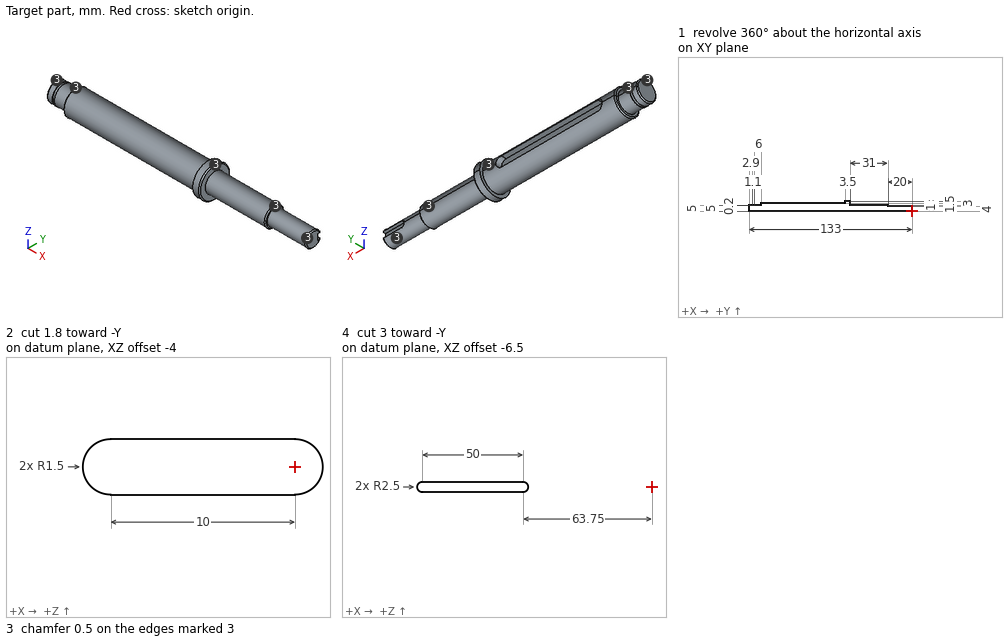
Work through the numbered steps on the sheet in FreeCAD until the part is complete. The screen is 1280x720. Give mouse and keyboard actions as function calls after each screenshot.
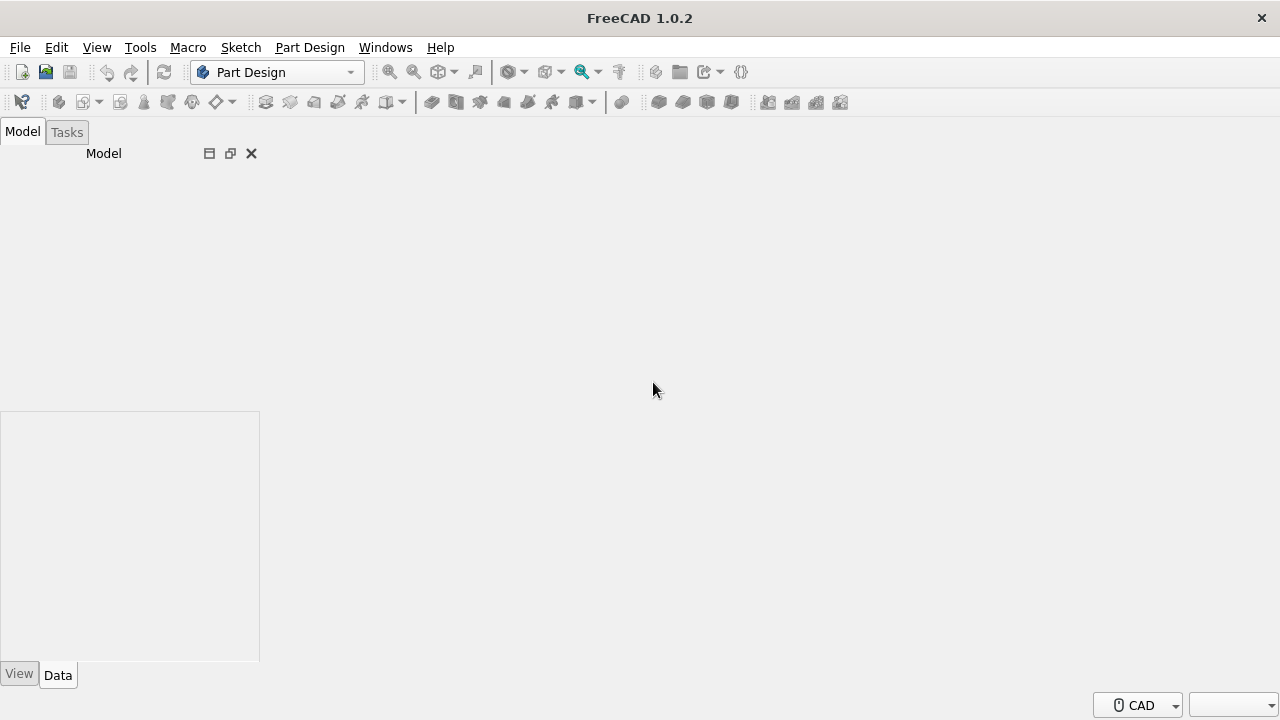
click(22, 72)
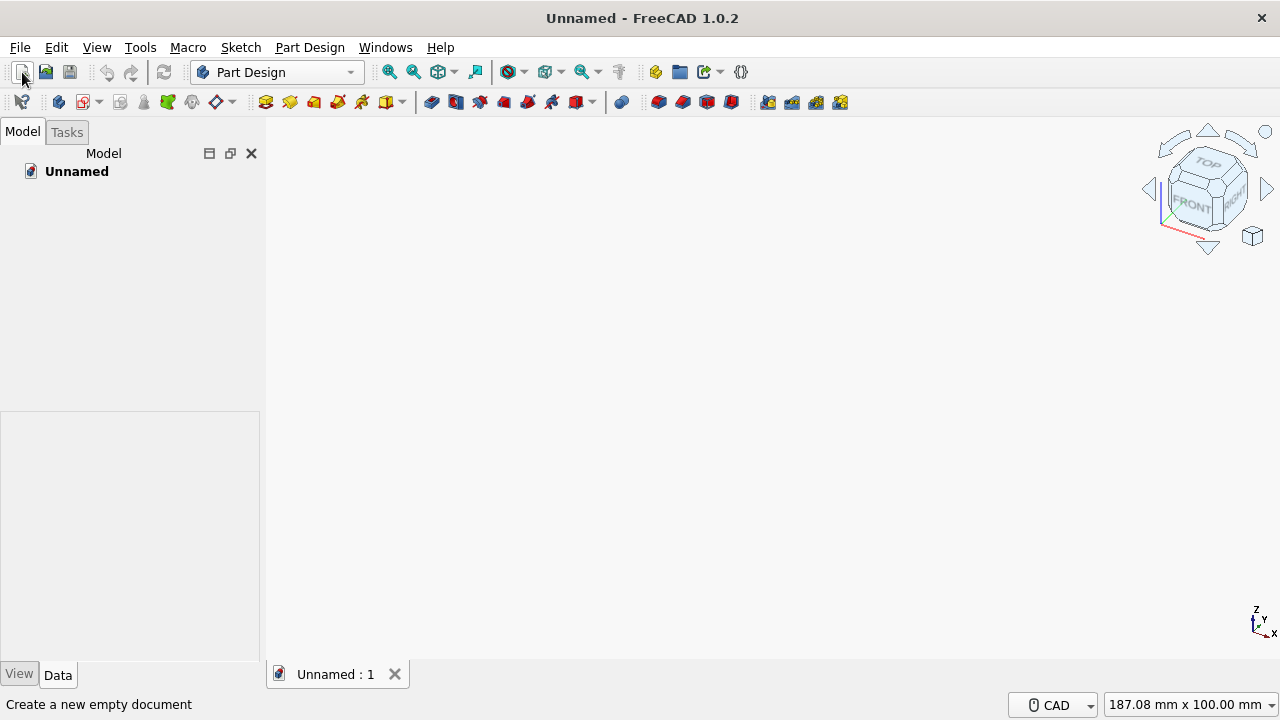
click(84, 102)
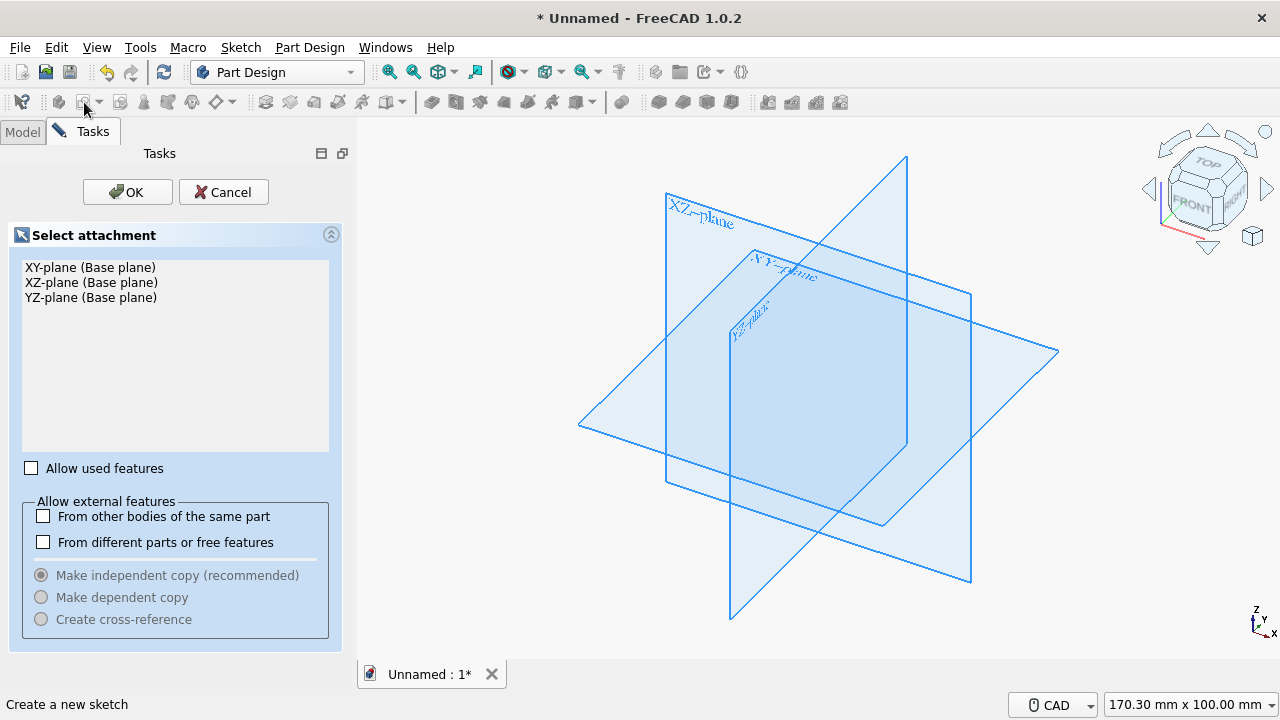
click(82, 268)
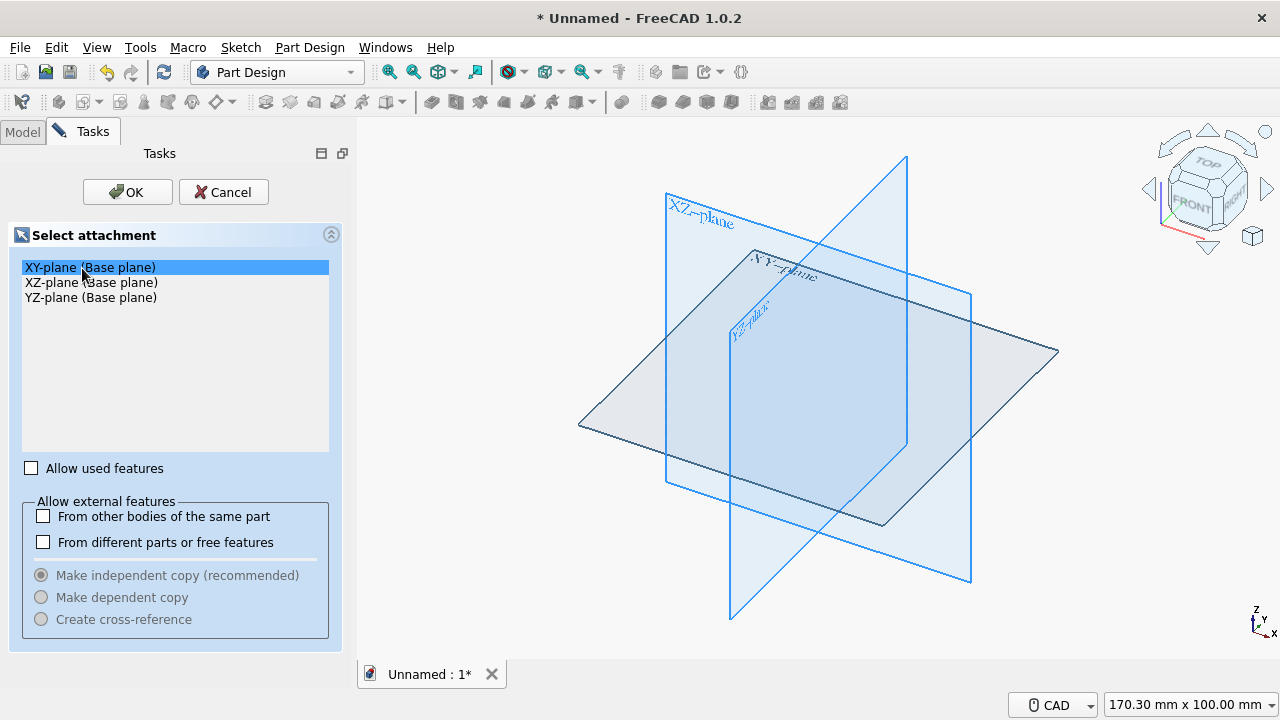
click(128, 192)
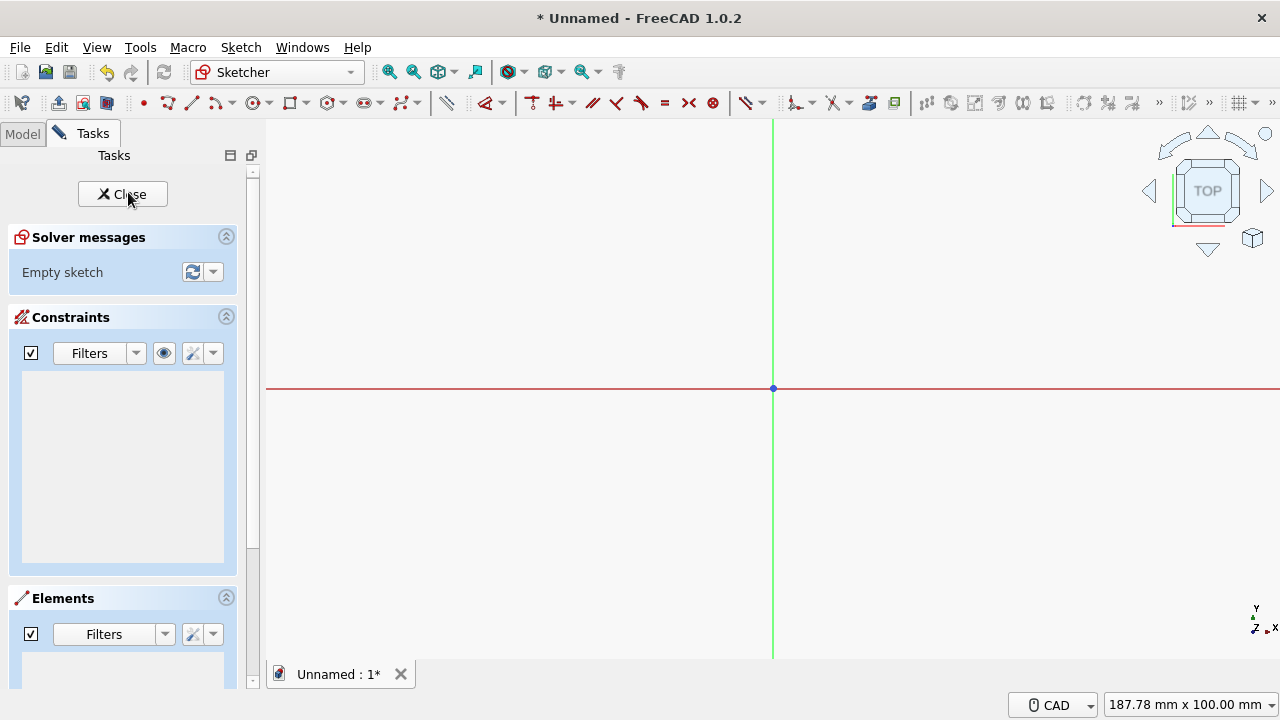
scroll(1115, 433, down, 2)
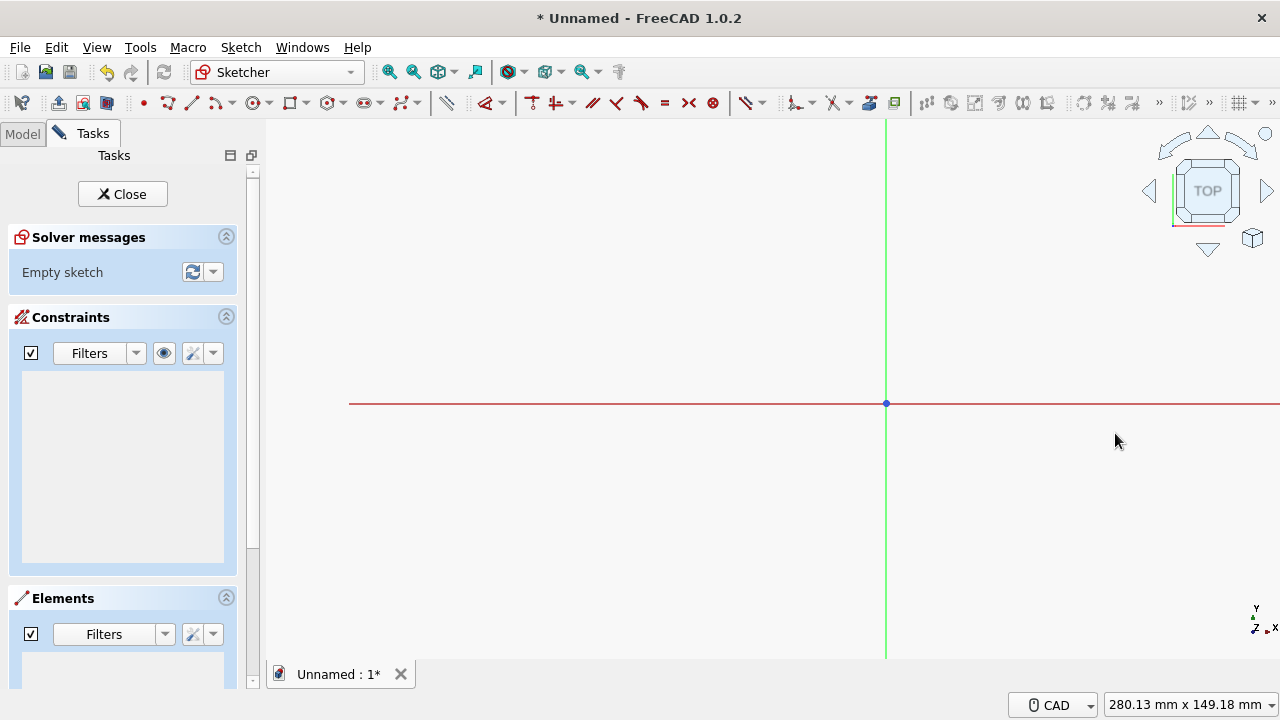
click(168, 104)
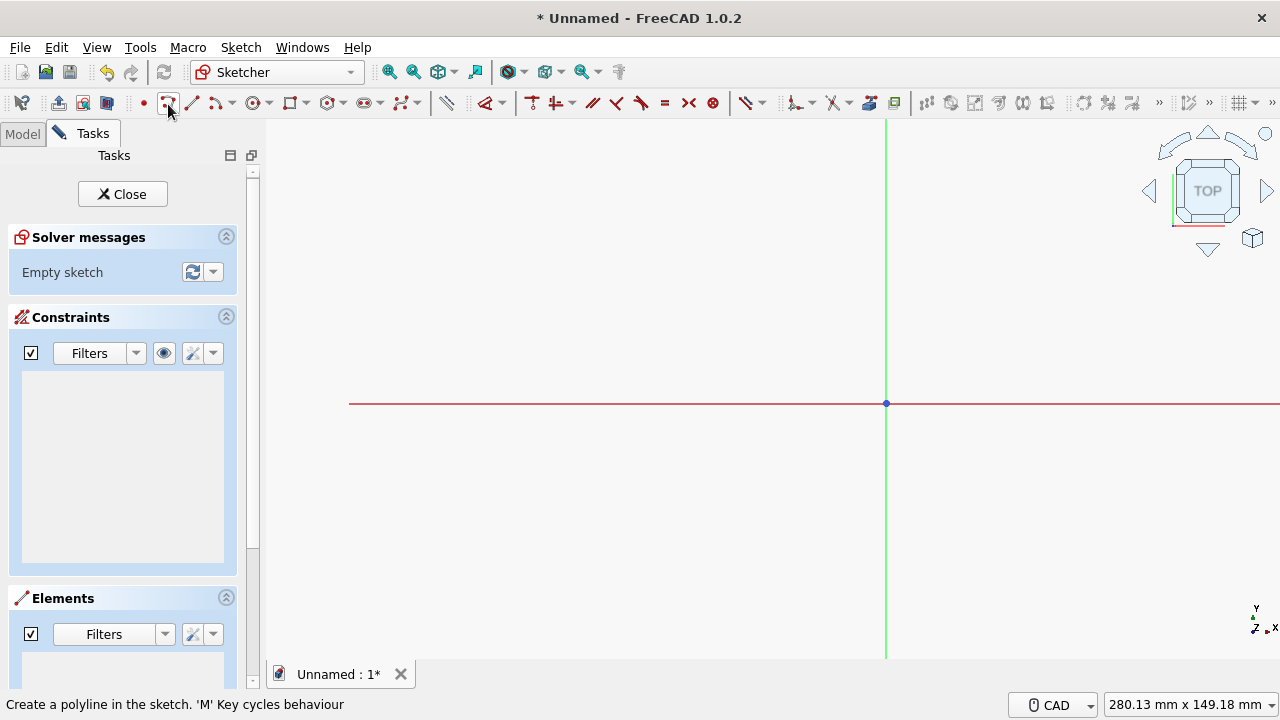
click(886, 404)
click(877, 389)
click(814, 389)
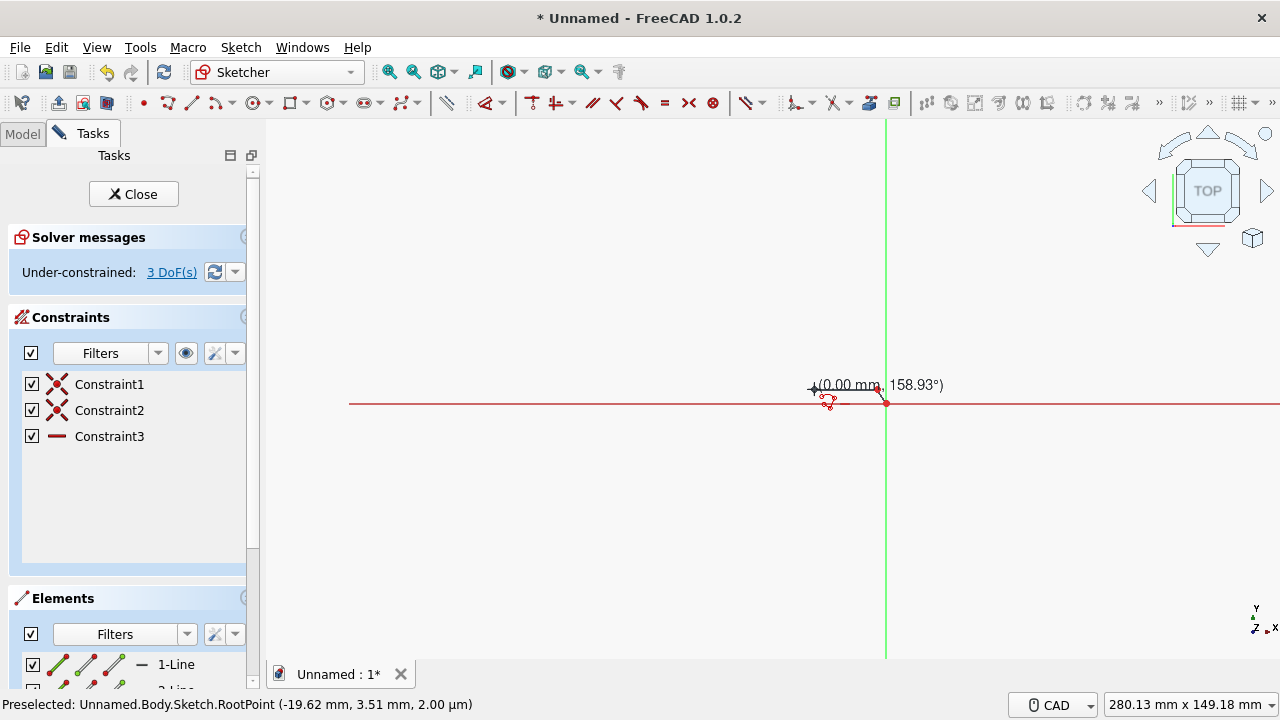
scroll(814, 386, up, 8)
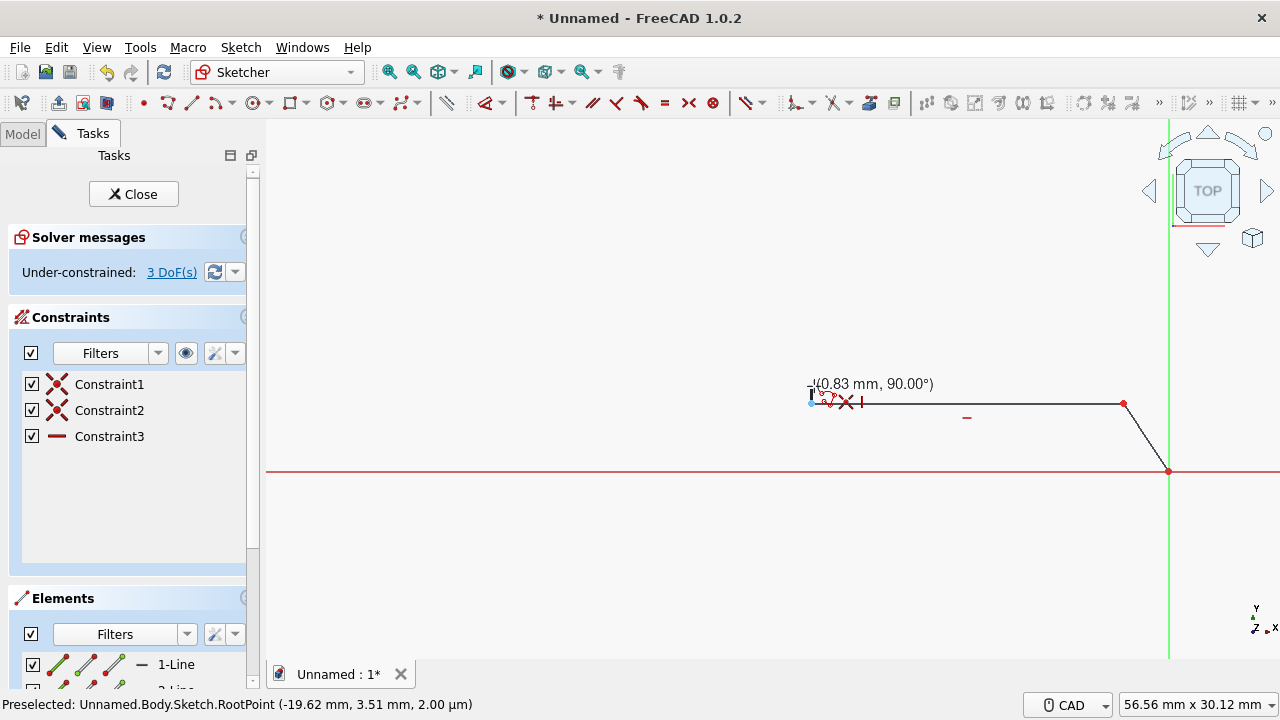
click(812, 382)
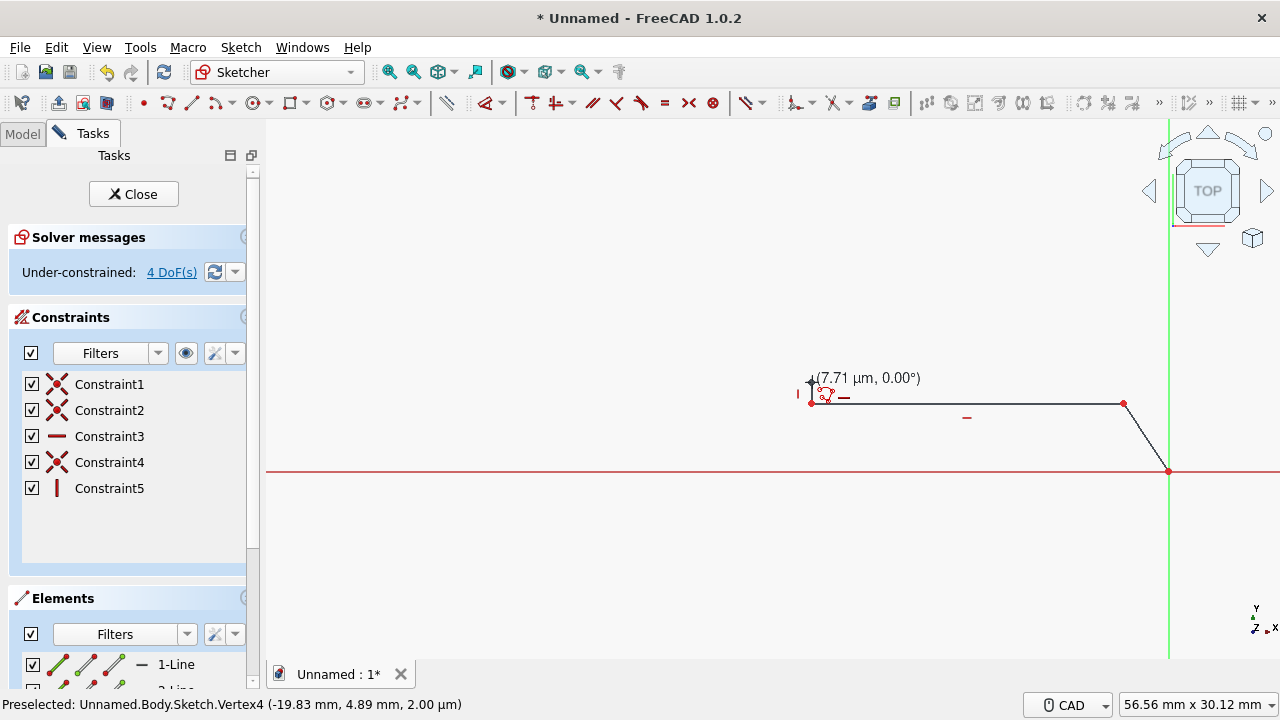
scroll(943, 385, down, 7)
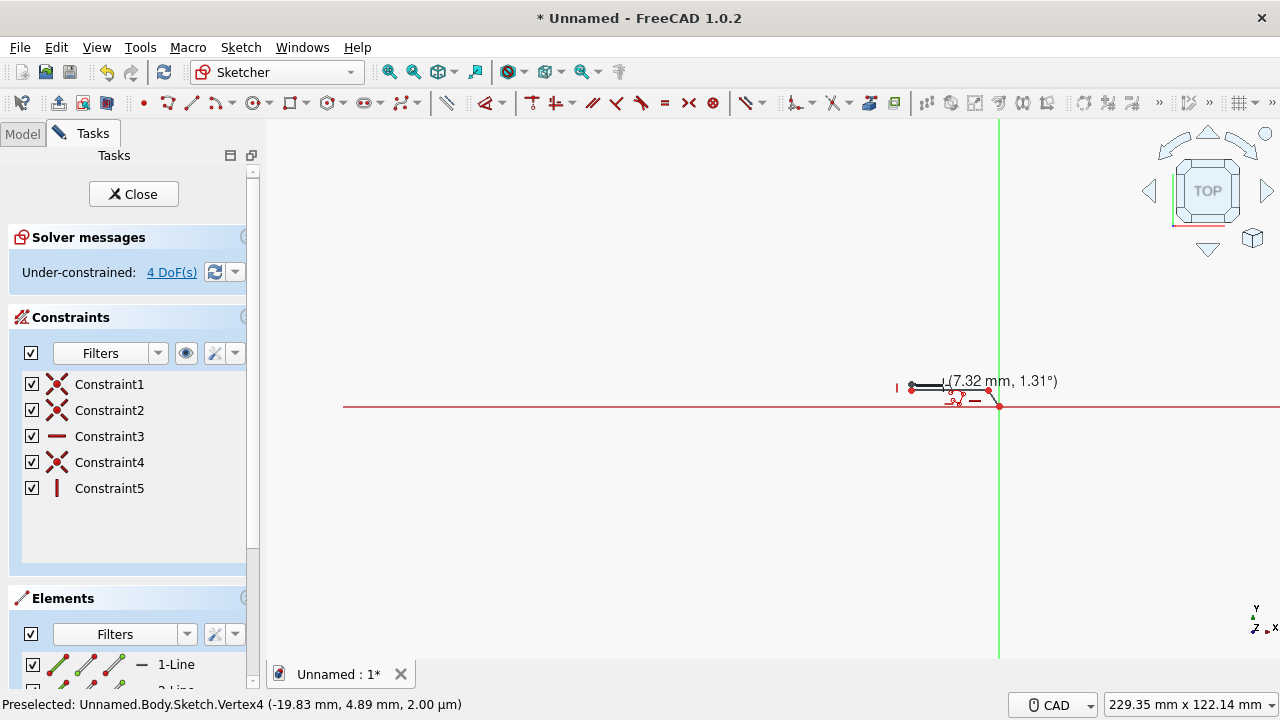
click(774, 385)
click(774, 371)
click(758, 371)